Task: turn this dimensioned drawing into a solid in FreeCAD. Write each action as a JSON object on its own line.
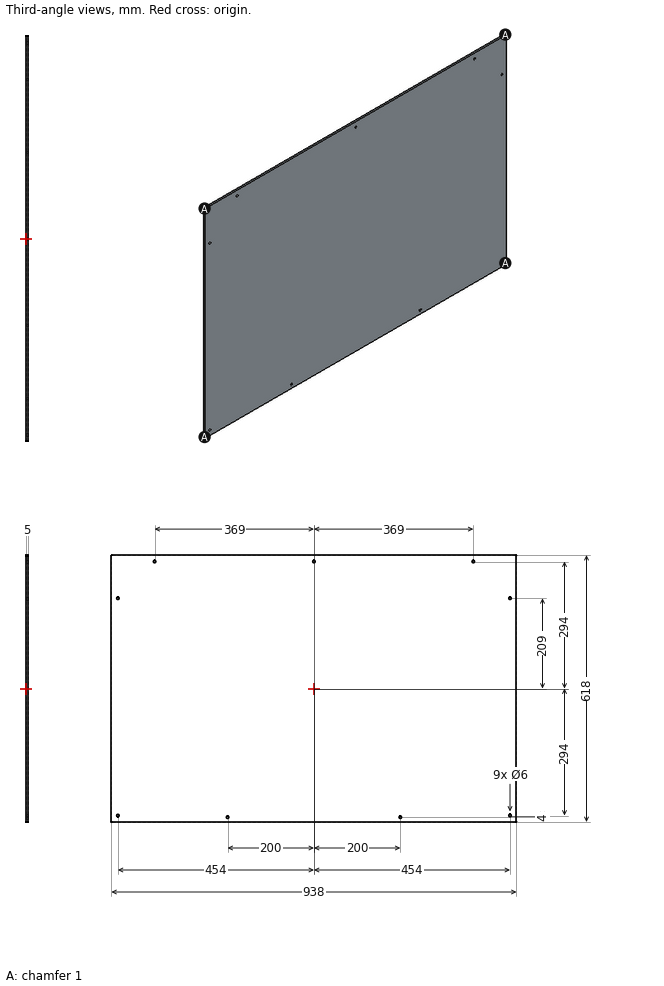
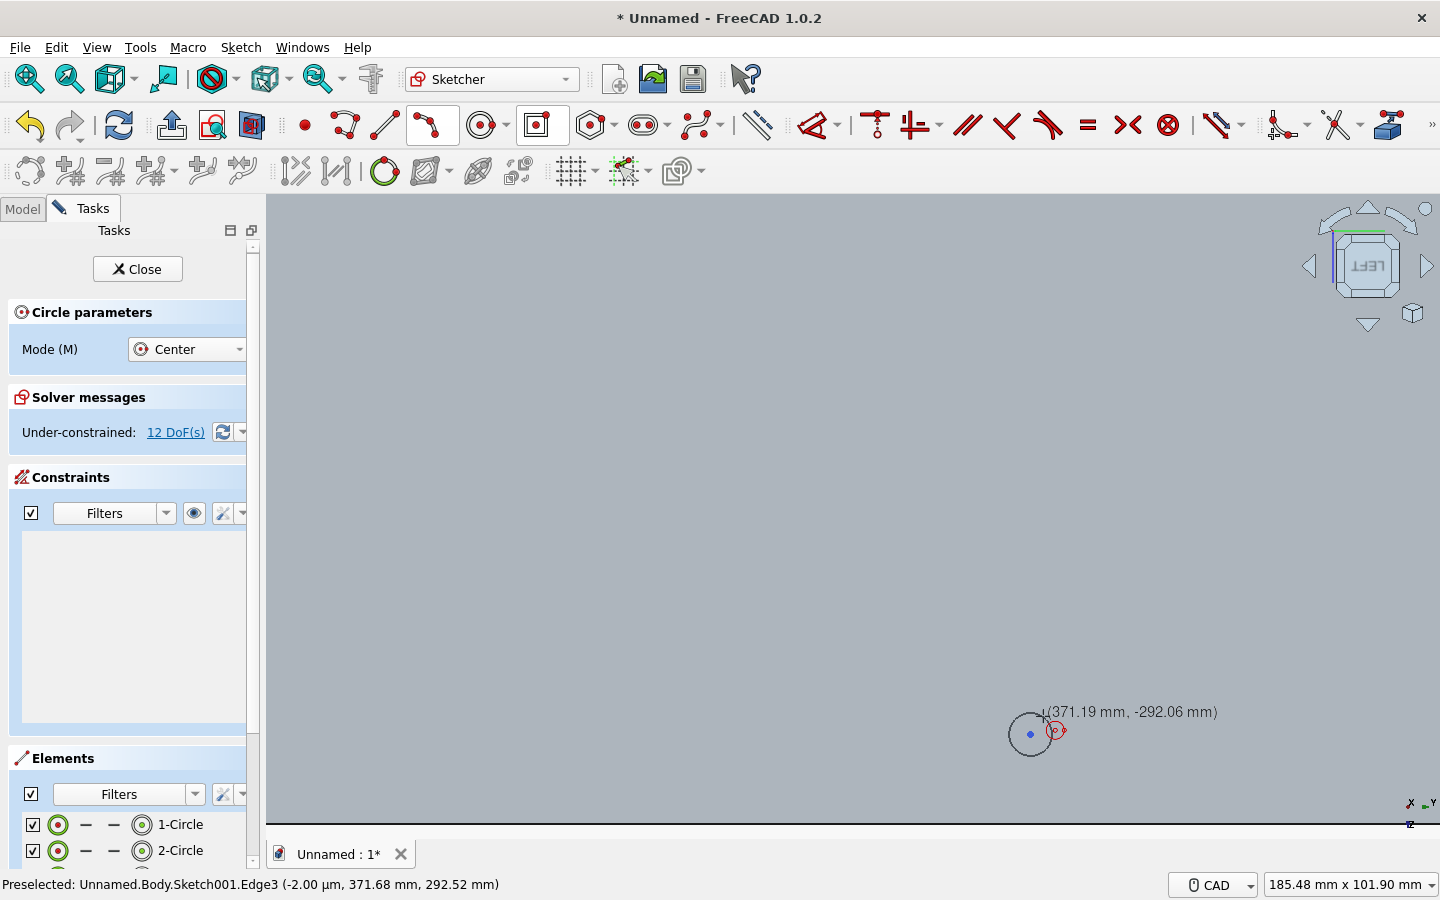
{"action": "scroll", "coordinate": [1045, 723], "scroll_direction": "down", "scroll_amount": 11}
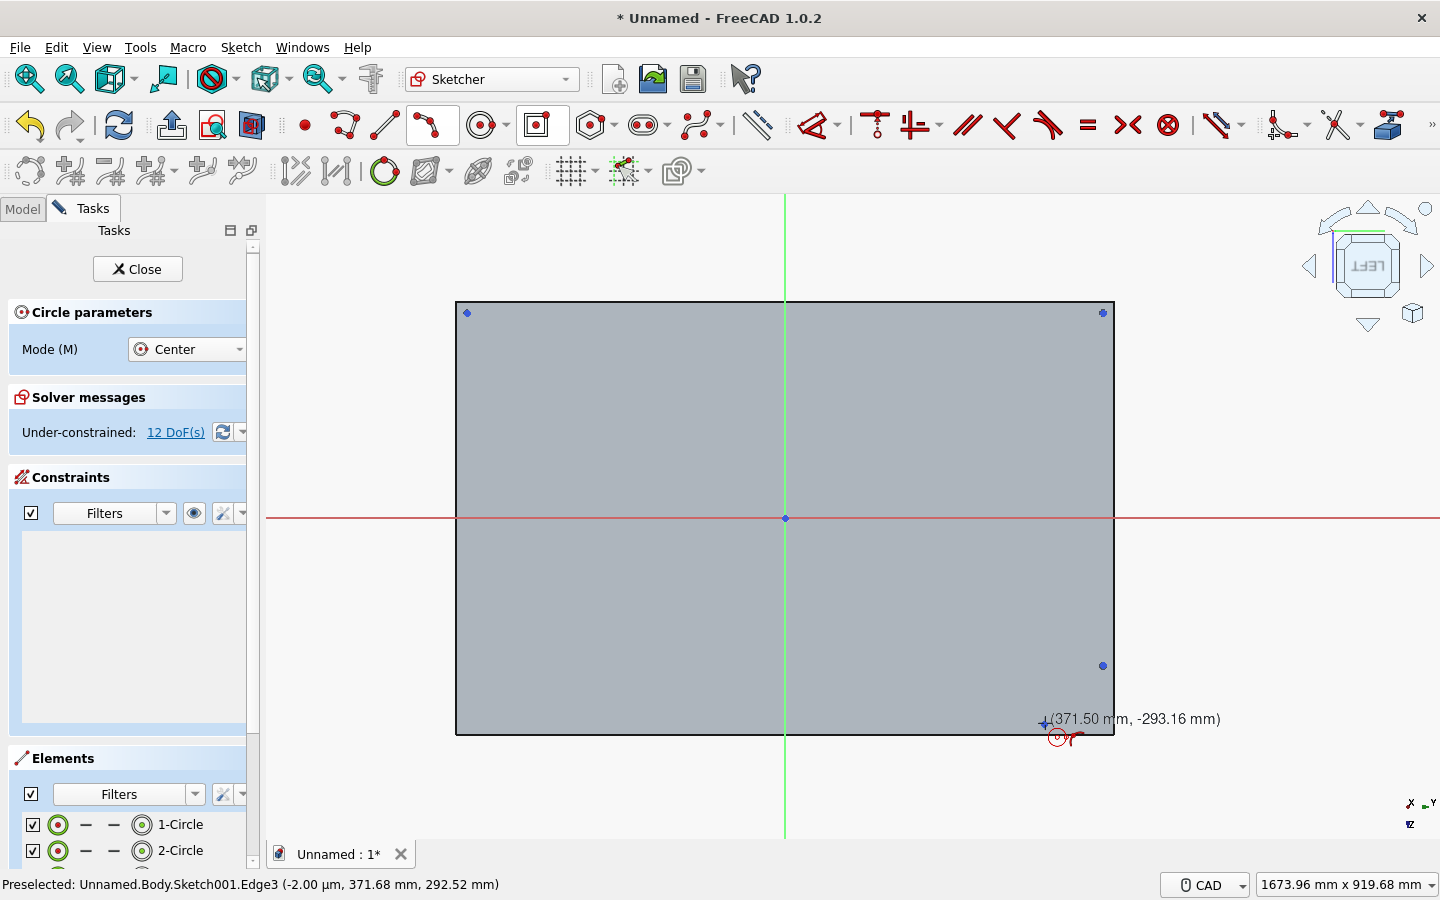
{"action": "scroll", "coordinate": [526, 724], "scroll_direction": "up", "scroll_amount": 12}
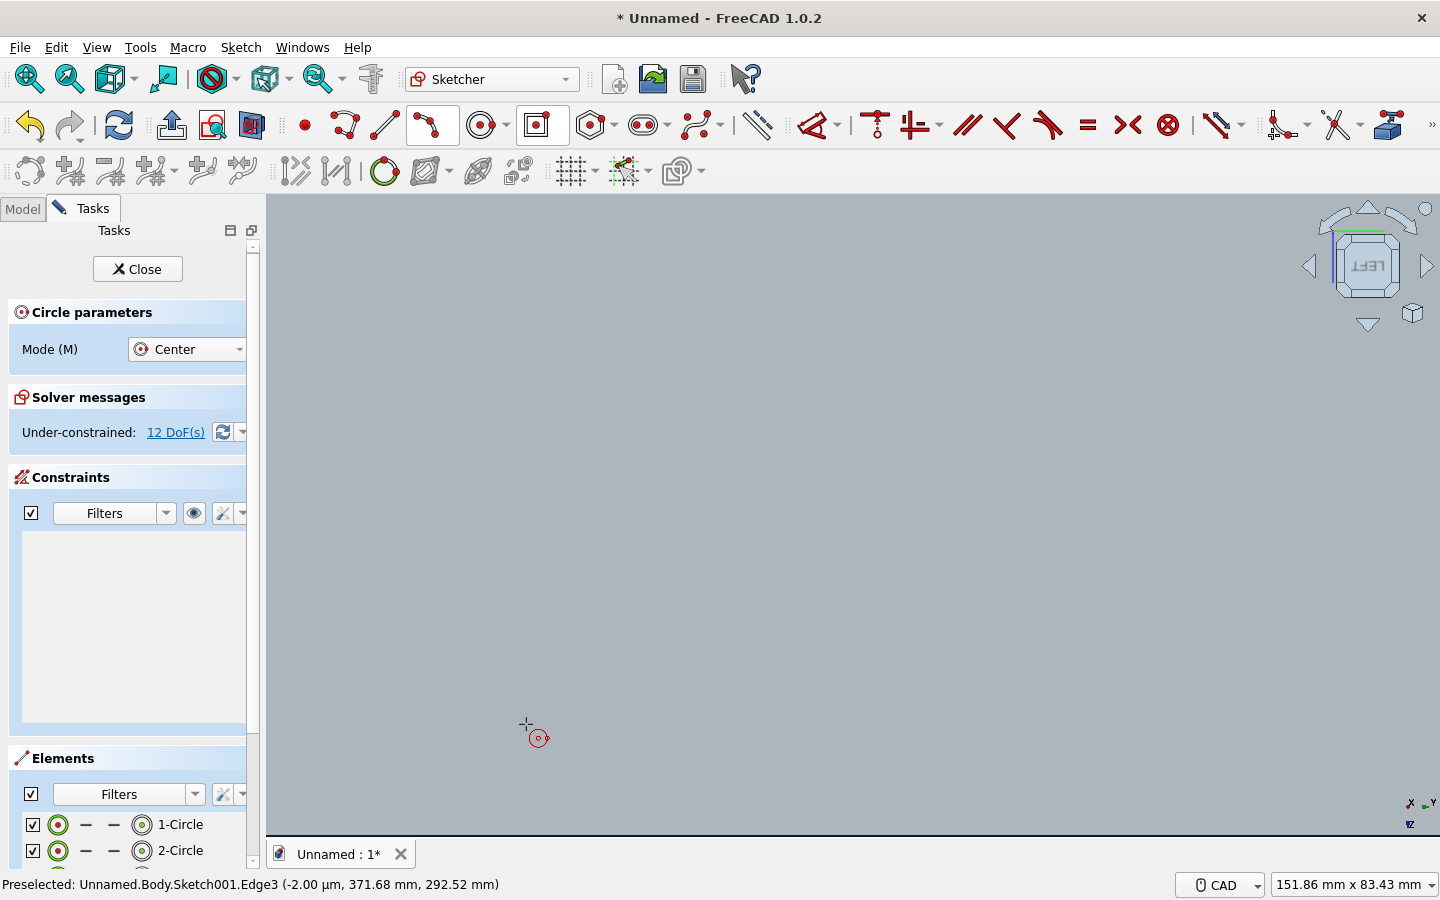
{"action": "scroll", "coordinate": [526, 724], "scroll_direction": "down", "scroll_amount": 12}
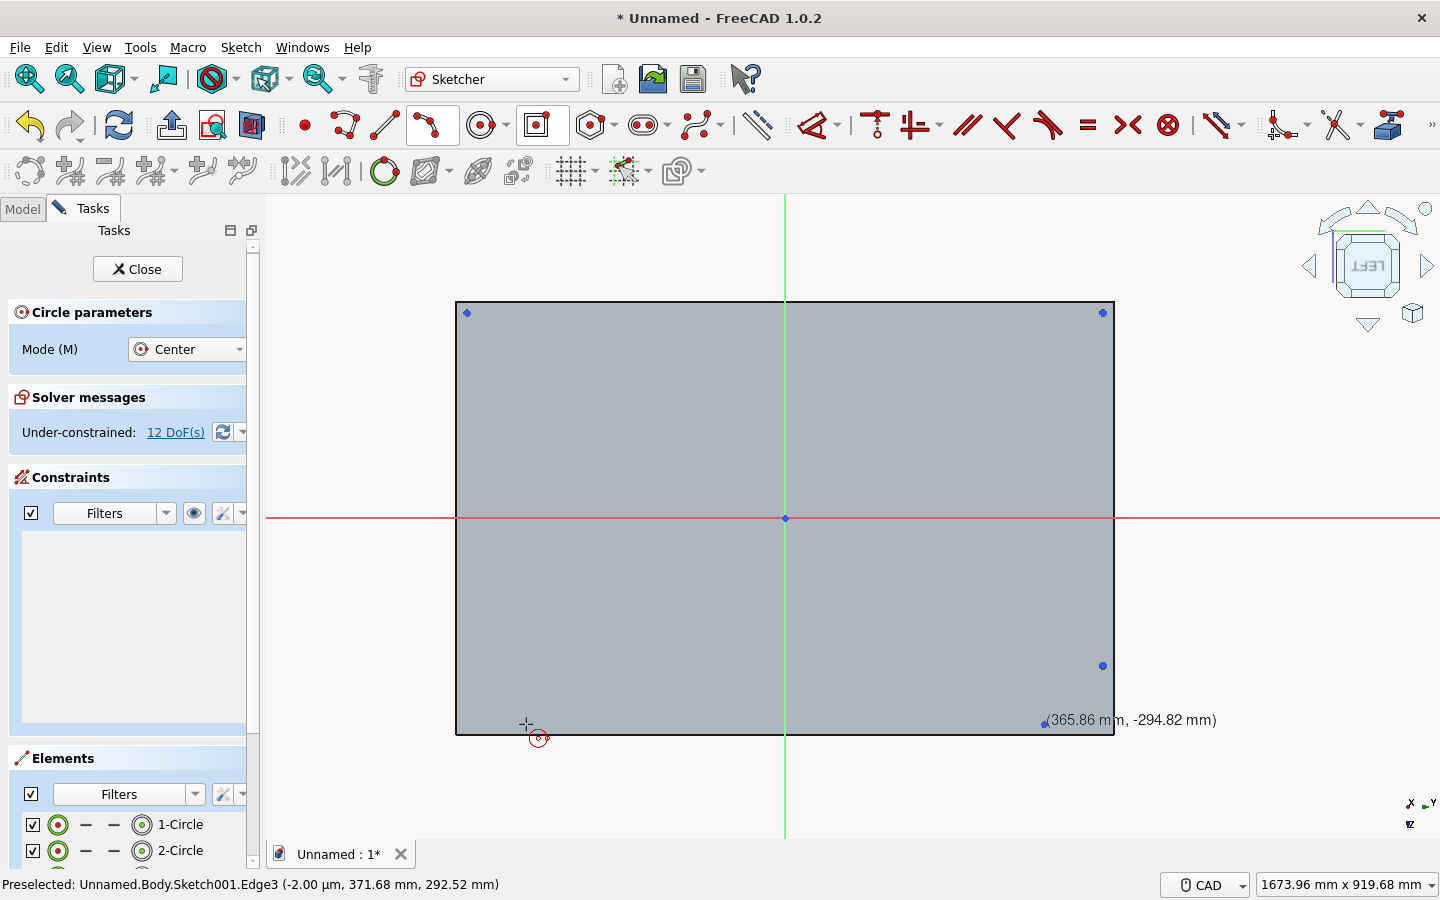
{"action": "left_click", "coordinate": [526, 724]}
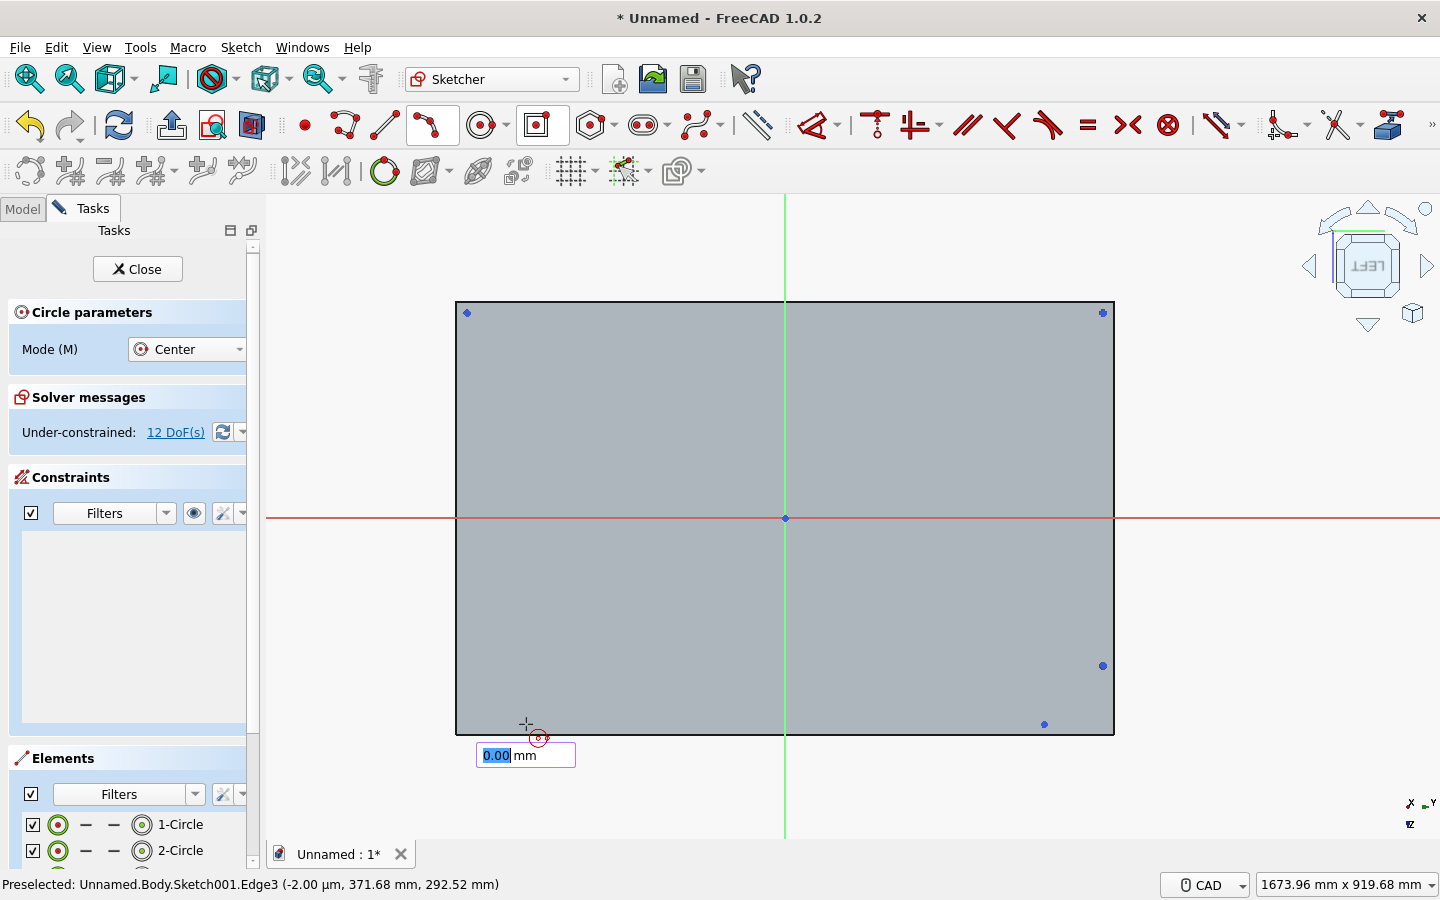
{"action": "scroll", "coordinate": [528, 723], "scroll_direction": "up", "scroll_amount": 11}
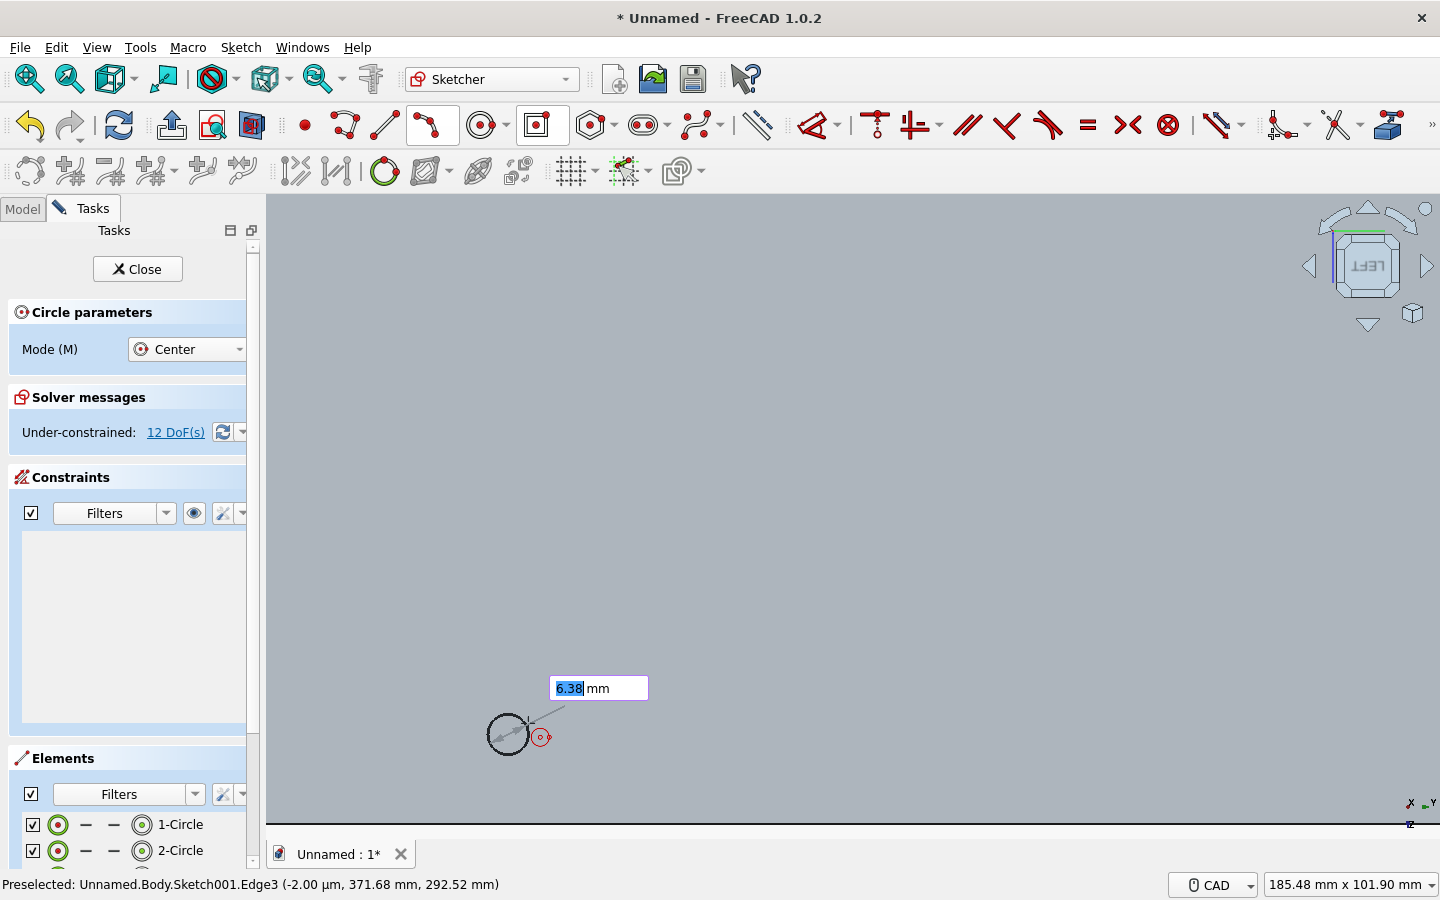
{"action": "left_click", "coordinate": [524, 716]}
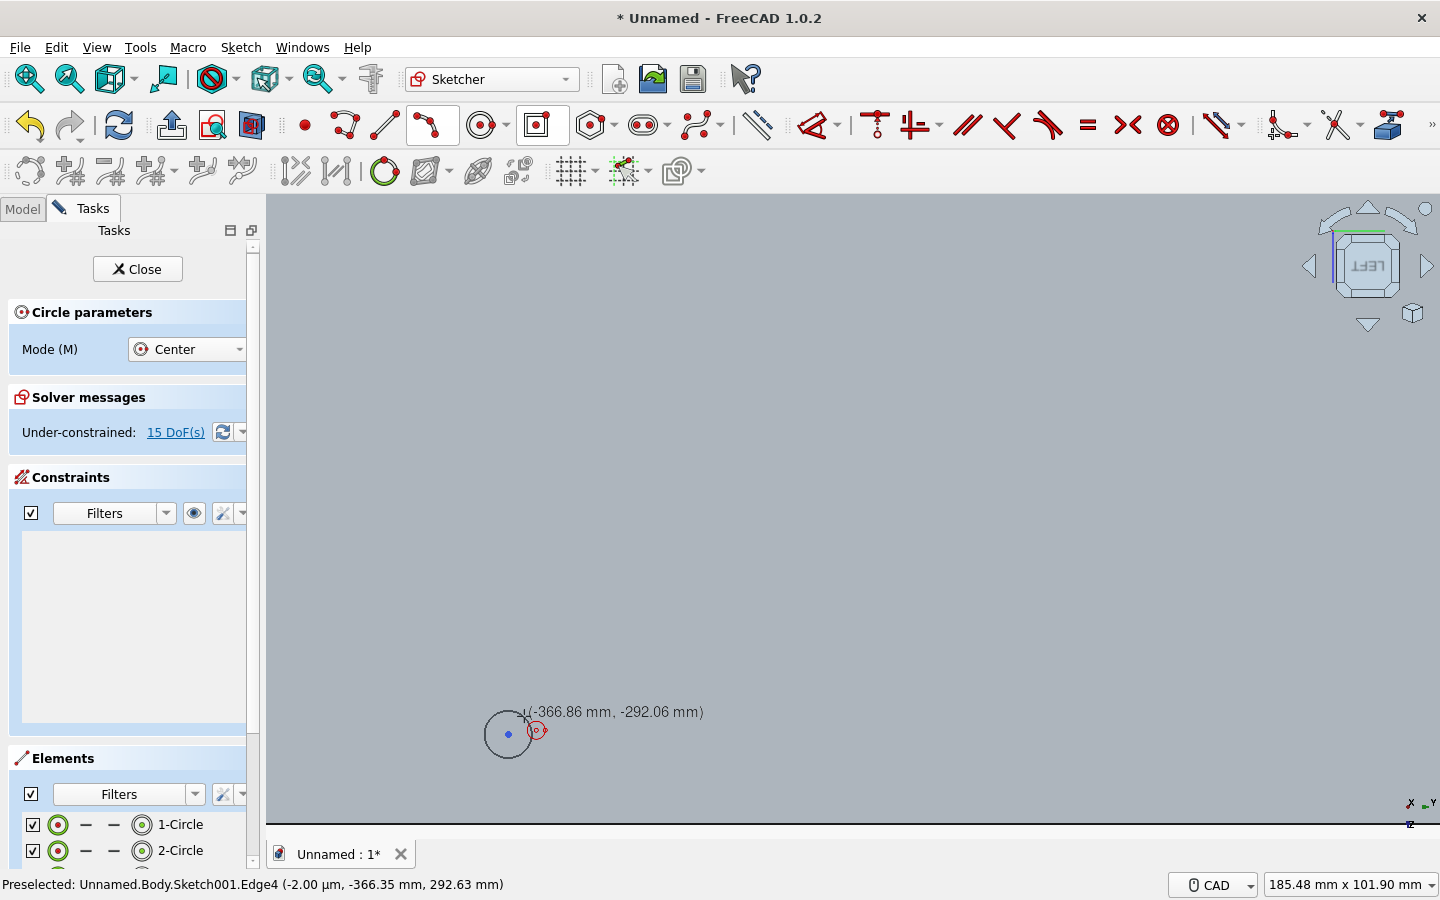
{"action": "scroll", "coordinate": [528, 723], "scroll_direction": "down", "scroll_amount": 11}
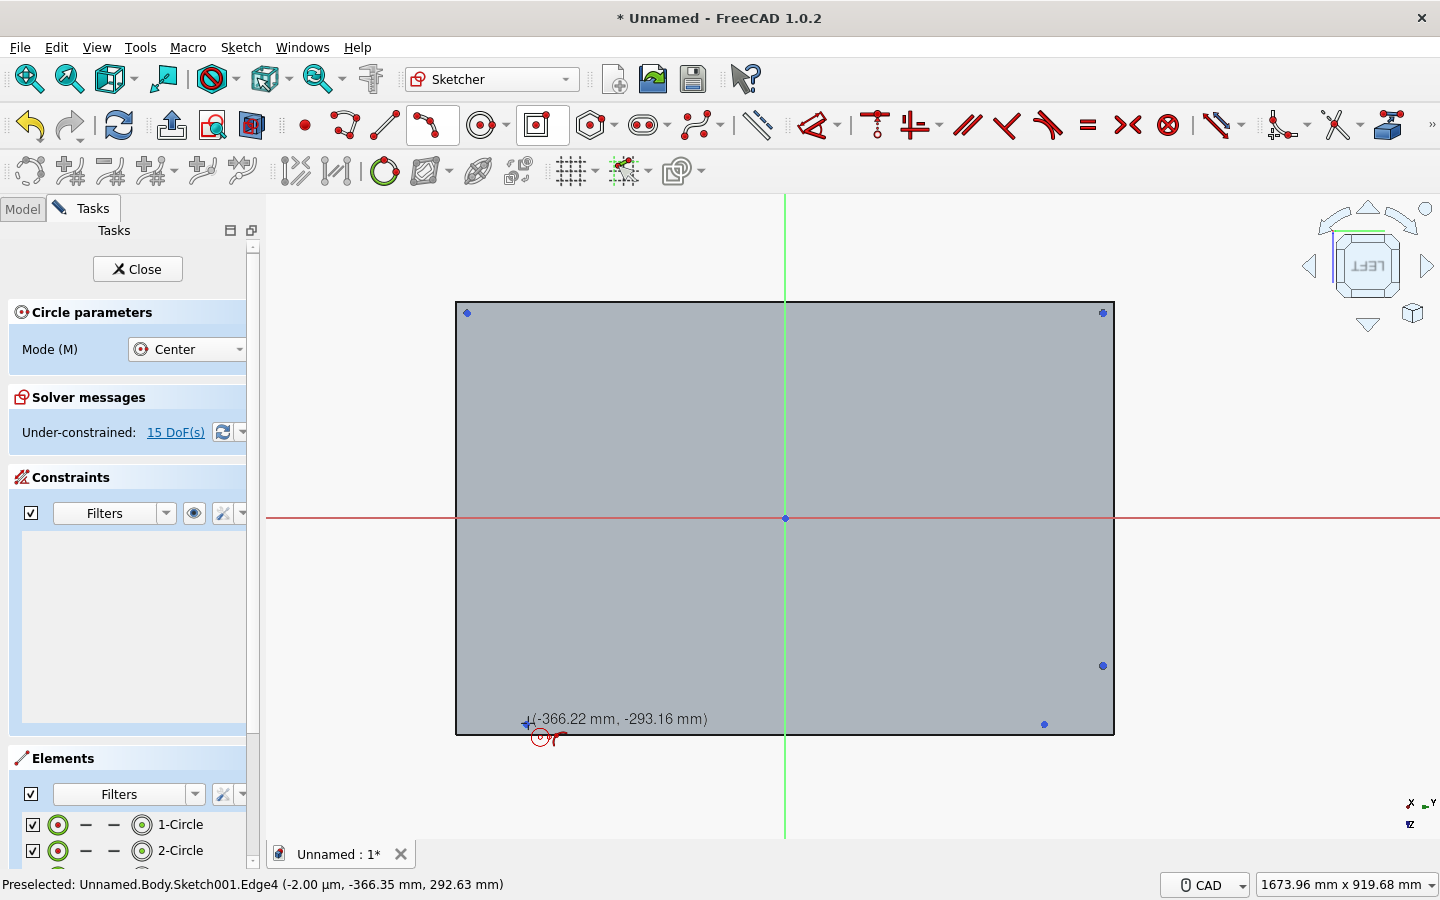
{"action": "scroll", "coordinate": [467, 665], "scroll_direction": "up", "scroll_amount": 12}